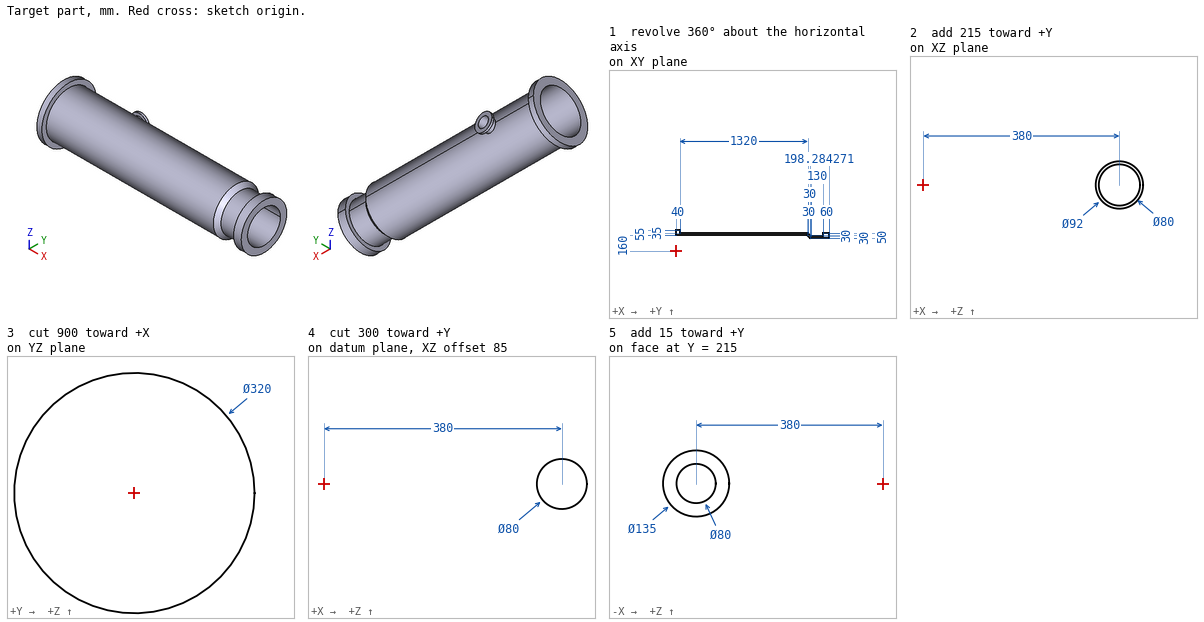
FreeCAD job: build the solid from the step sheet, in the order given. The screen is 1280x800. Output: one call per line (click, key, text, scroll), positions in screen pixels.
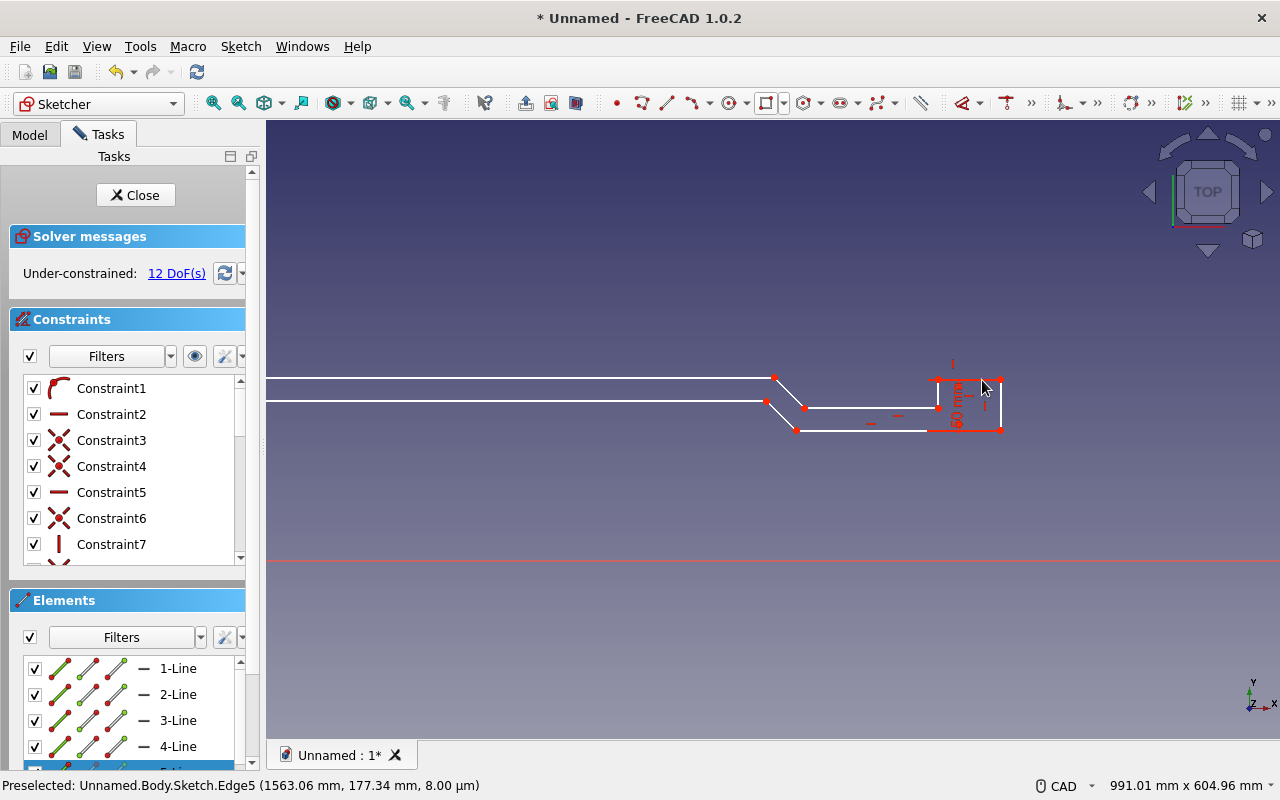
key(l)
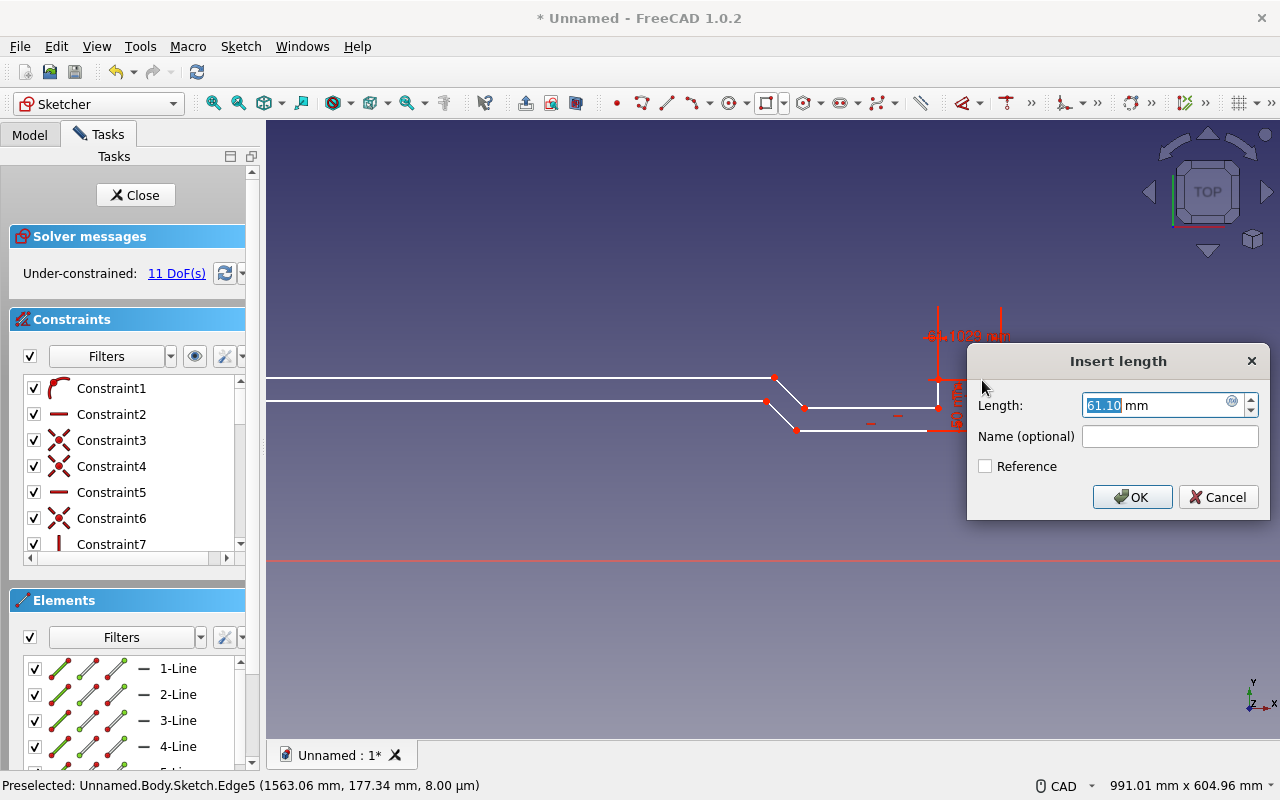
text(60)
key(Return)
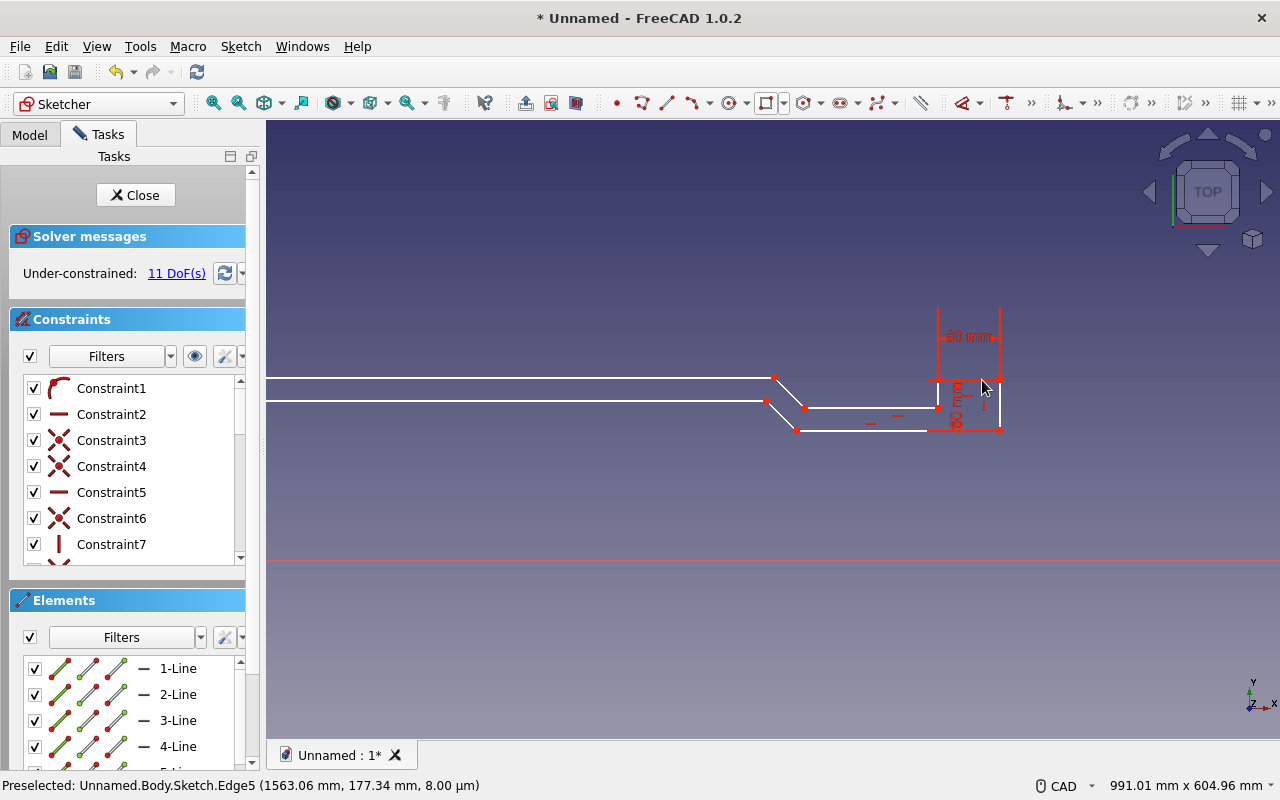
scroll(938, 391, up, 2)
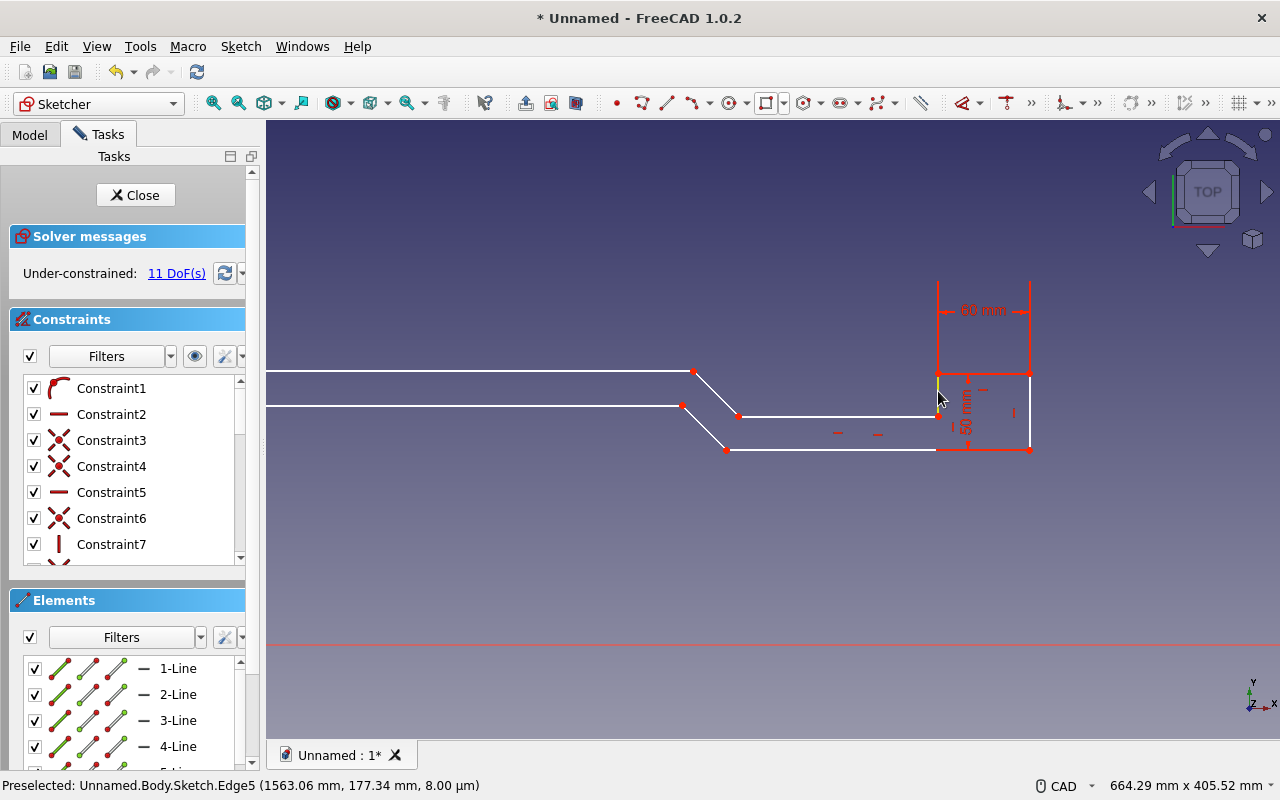
click(938, 391)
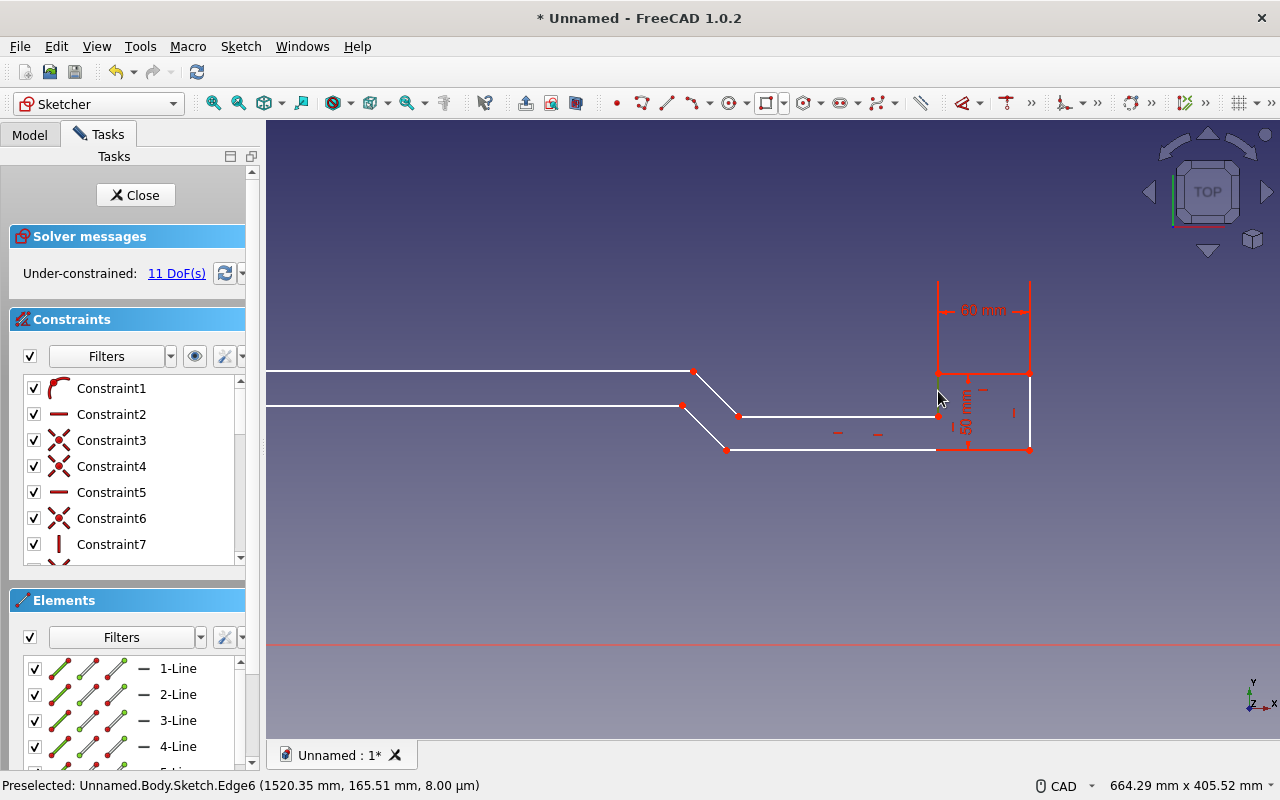
key(i)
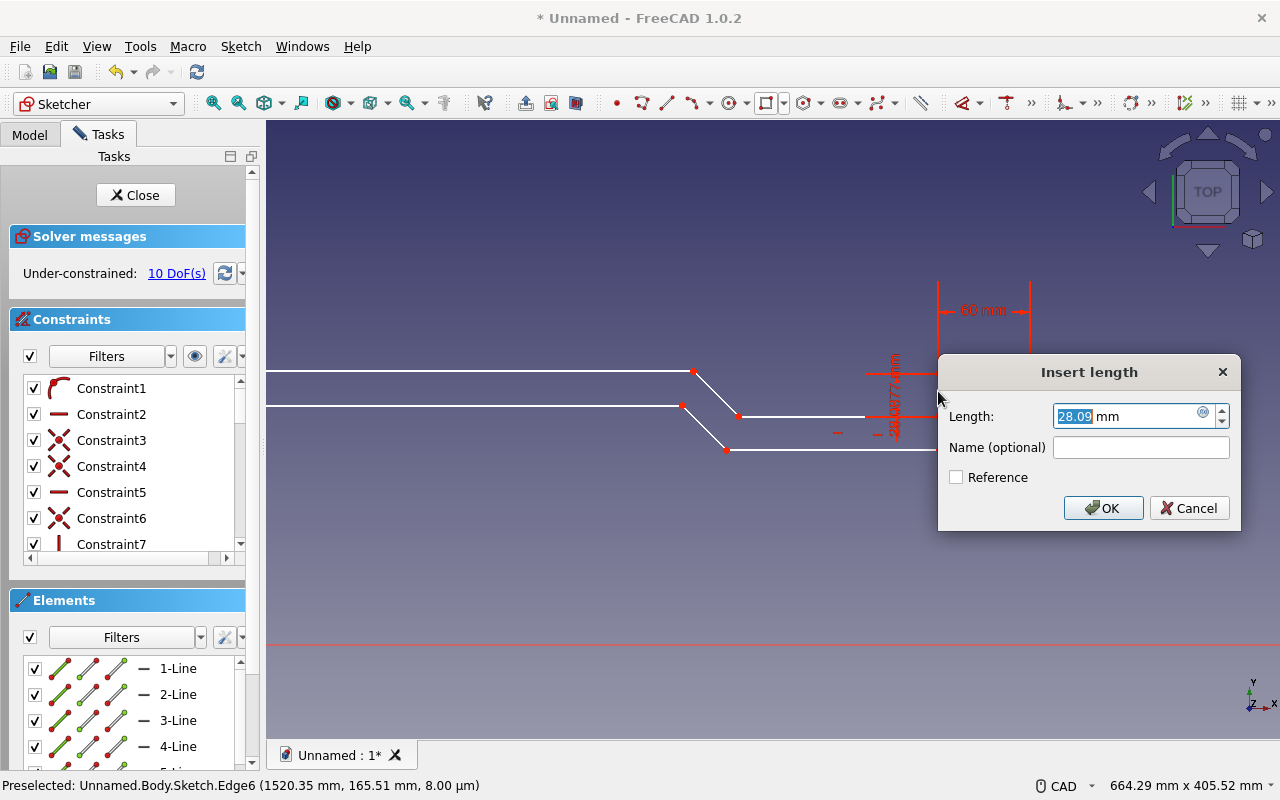
text(30)
key(Return)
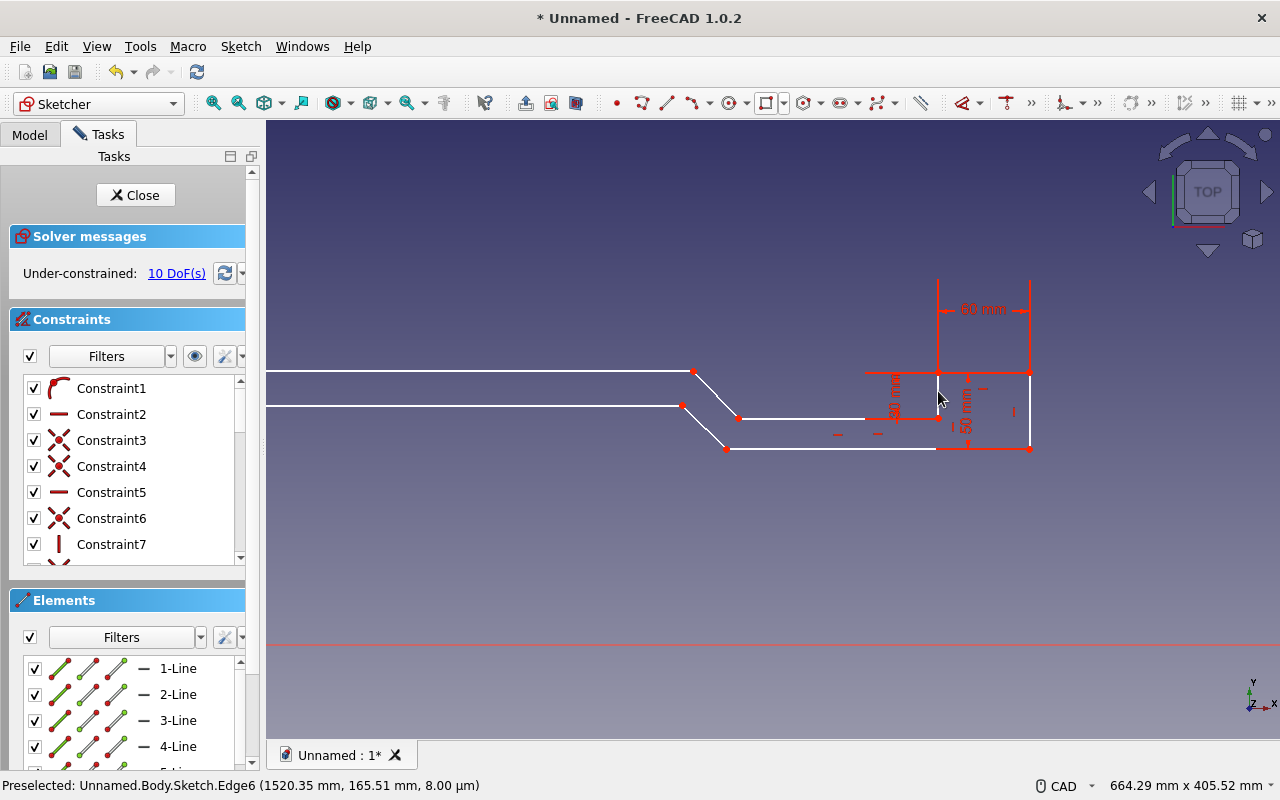
scroll(993, 413, down, 7)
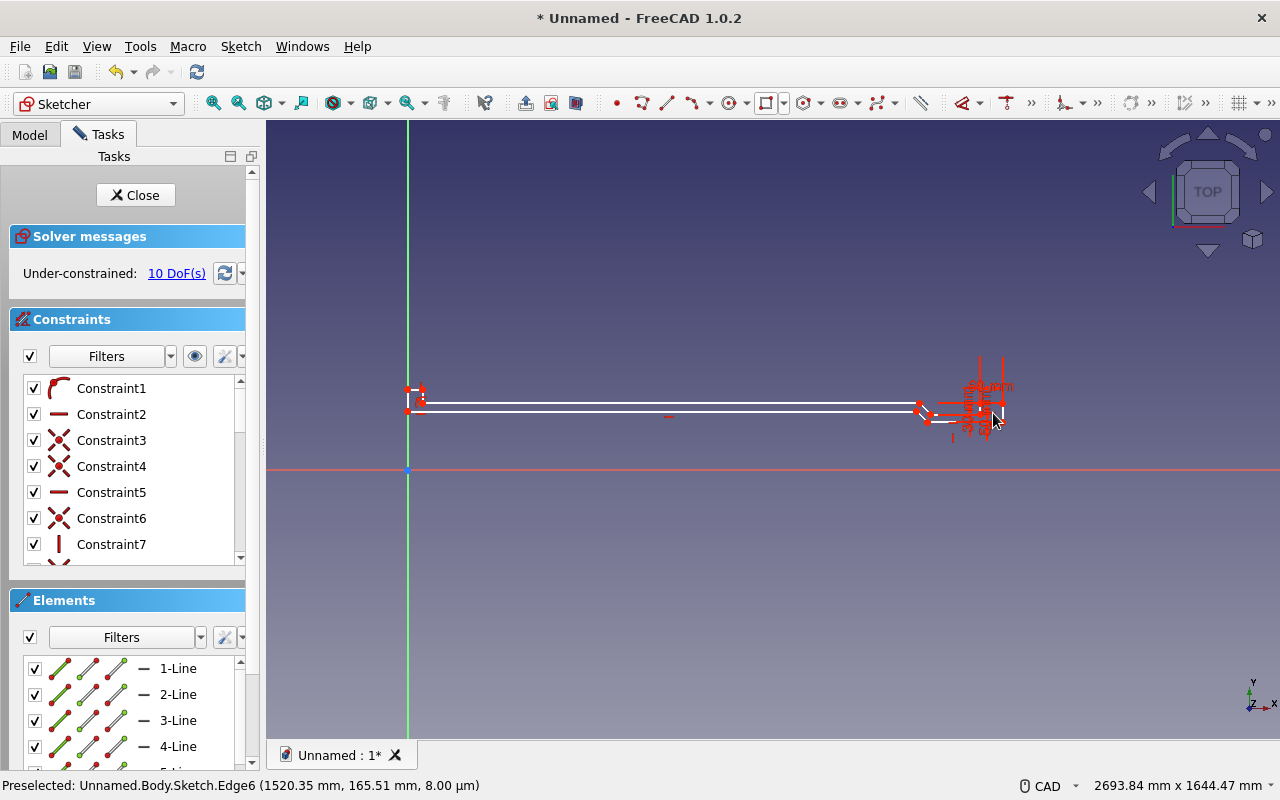
scroll(423, 399, up, 7)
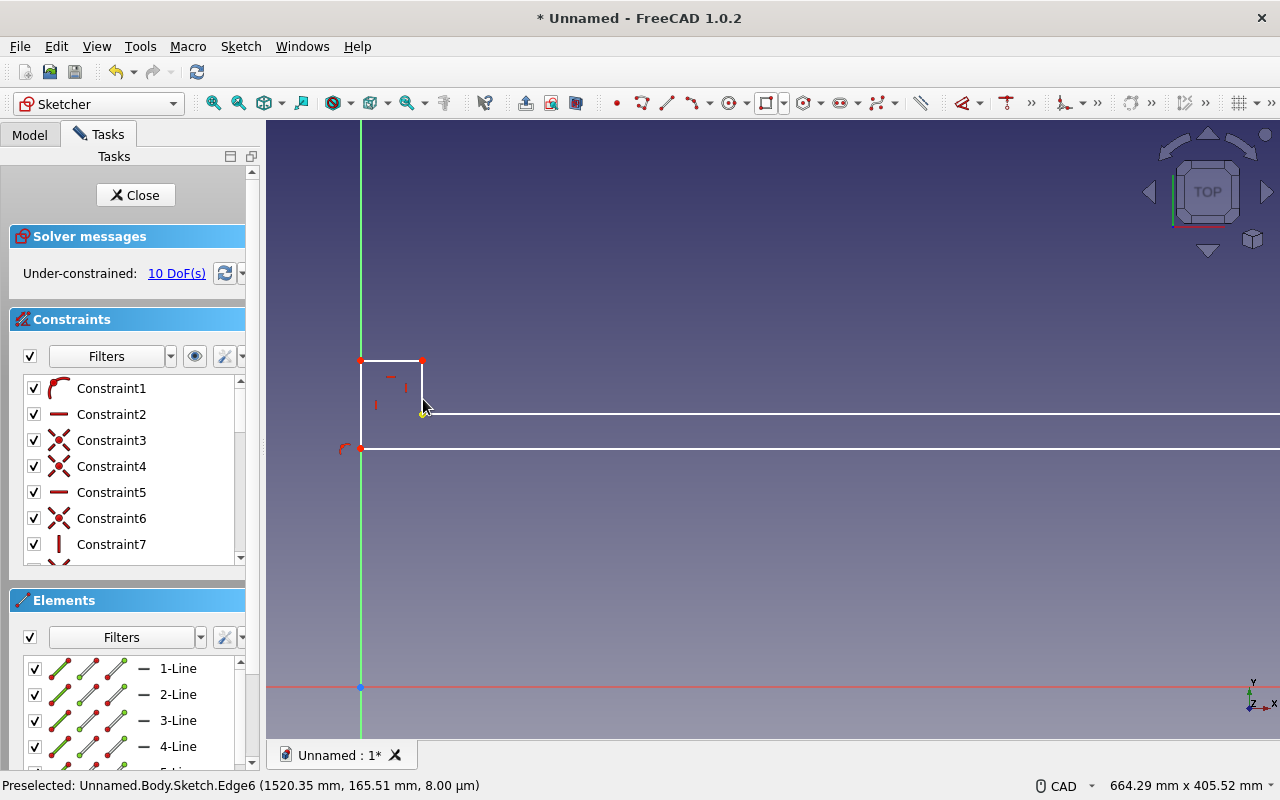
click(422, 398)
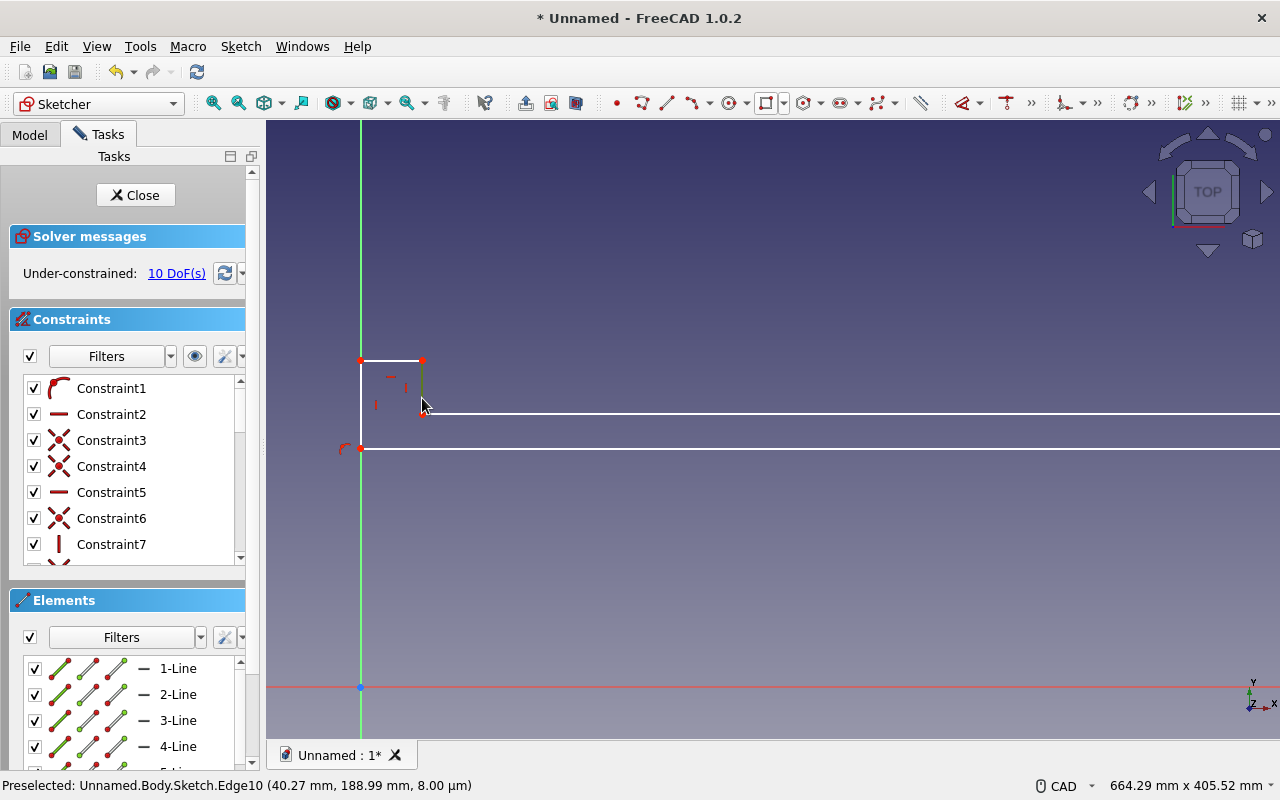
key(i)